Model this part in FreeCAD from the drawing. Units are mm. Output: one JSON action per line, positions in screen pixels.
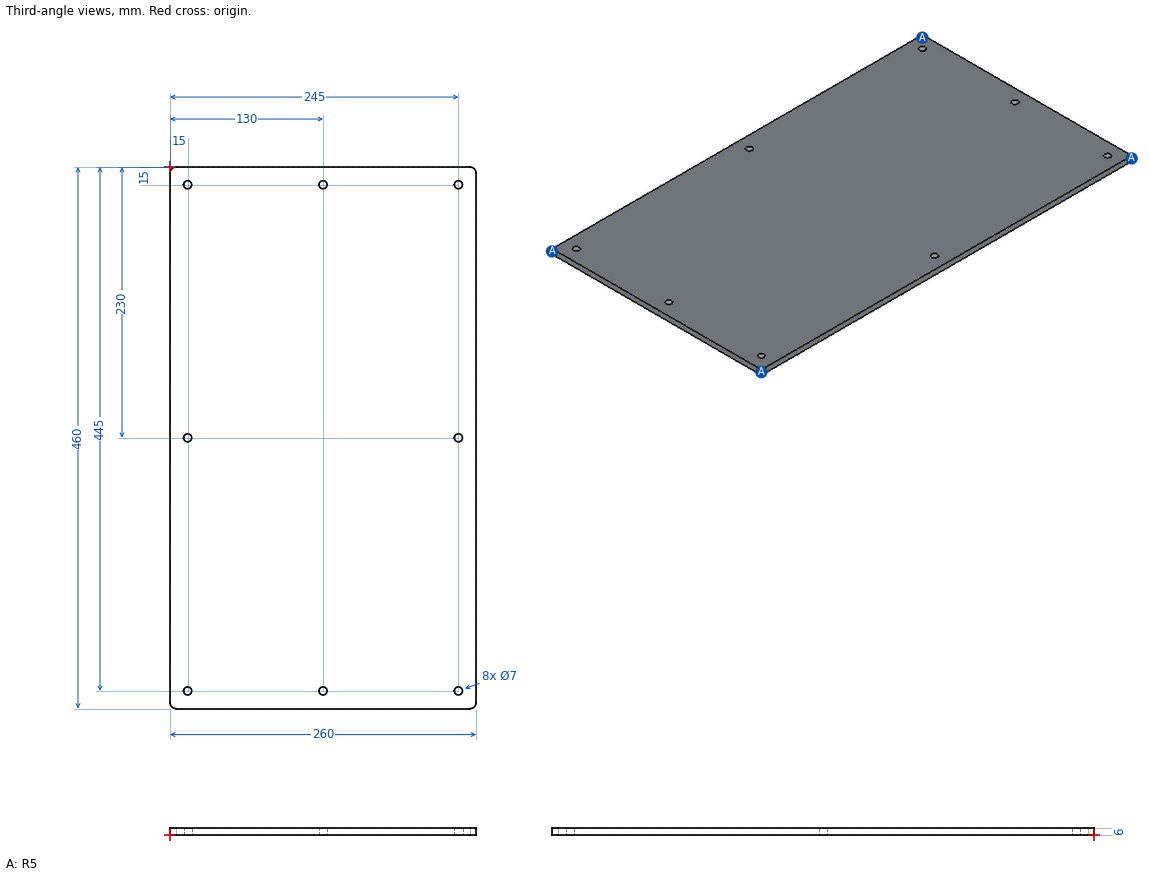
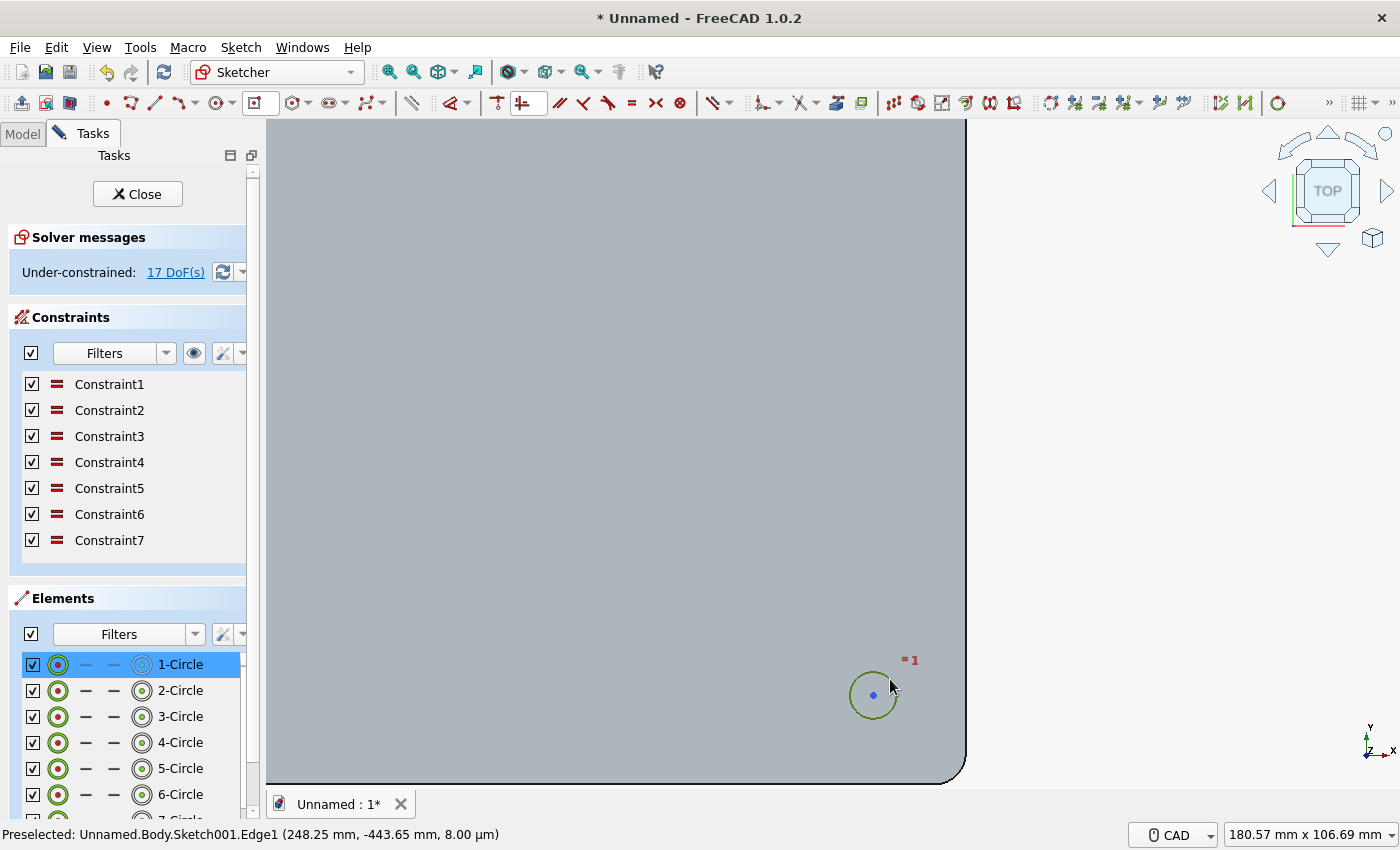
{"action": "key", "text": "k o"}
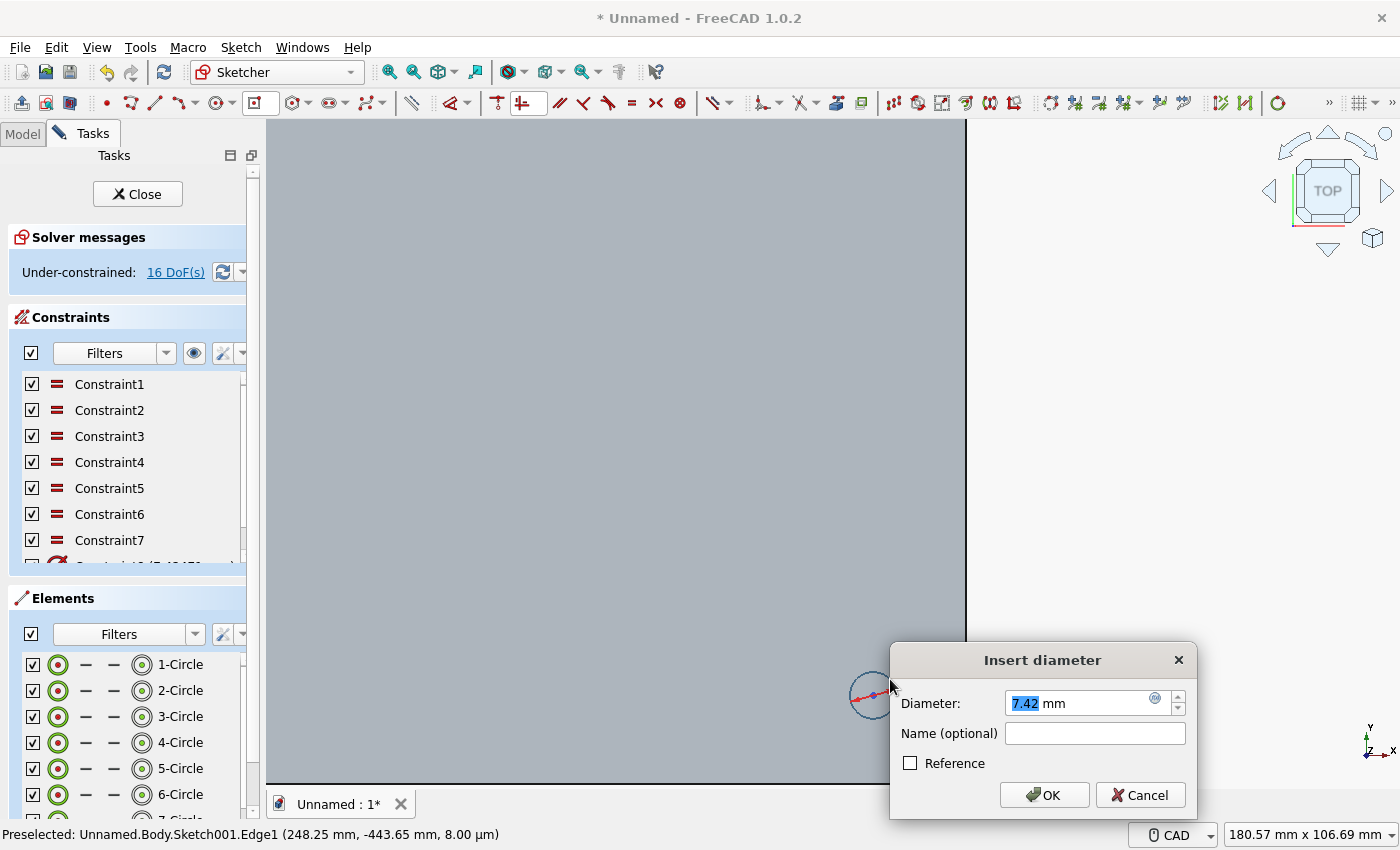
{"action": "type", "text": "7"}
{"action": "key", "text": "Return"}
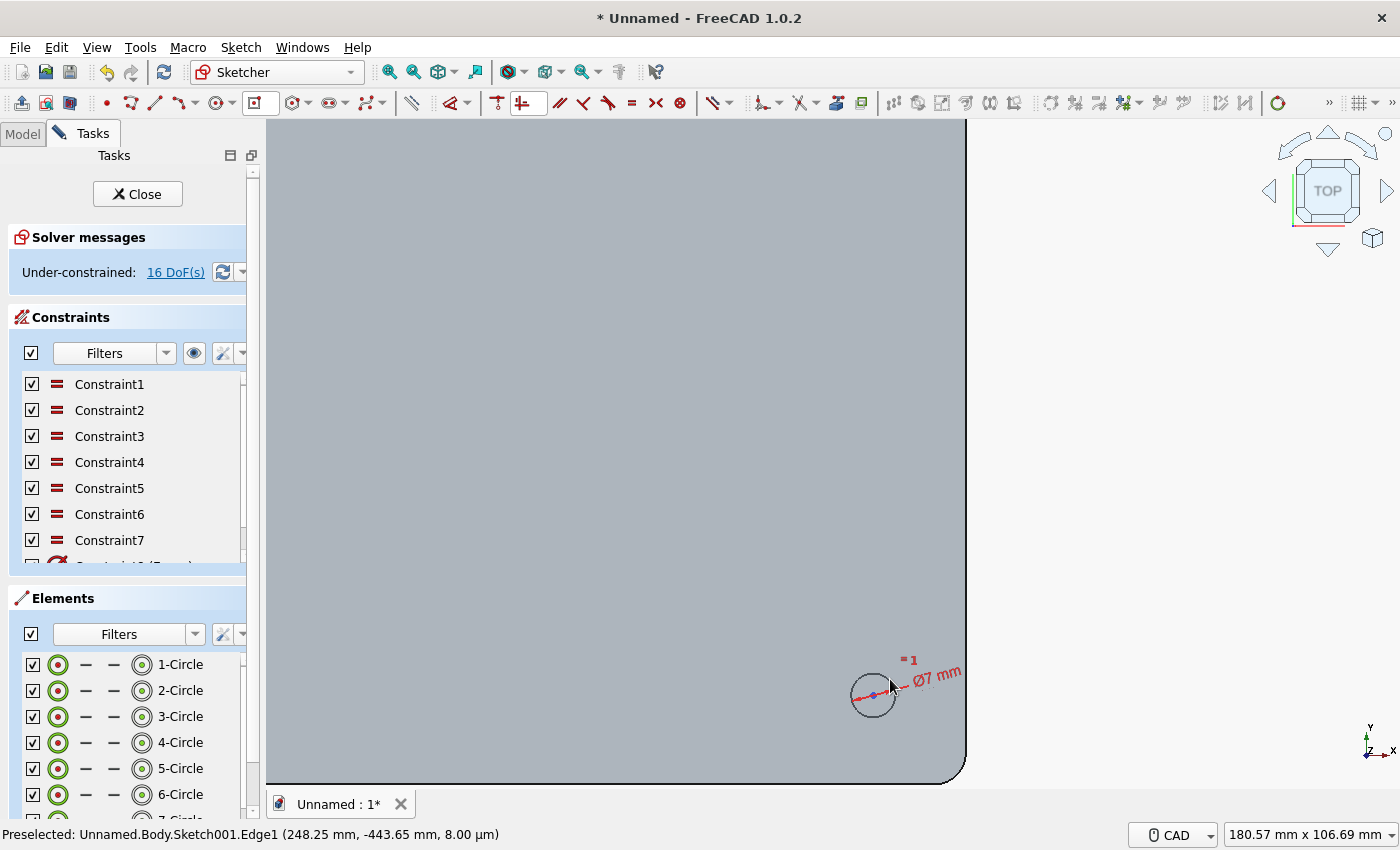
{"action": "scroll", "coordinate": [893, 682], "scroll_direction": "down", "scroll_amount": 9}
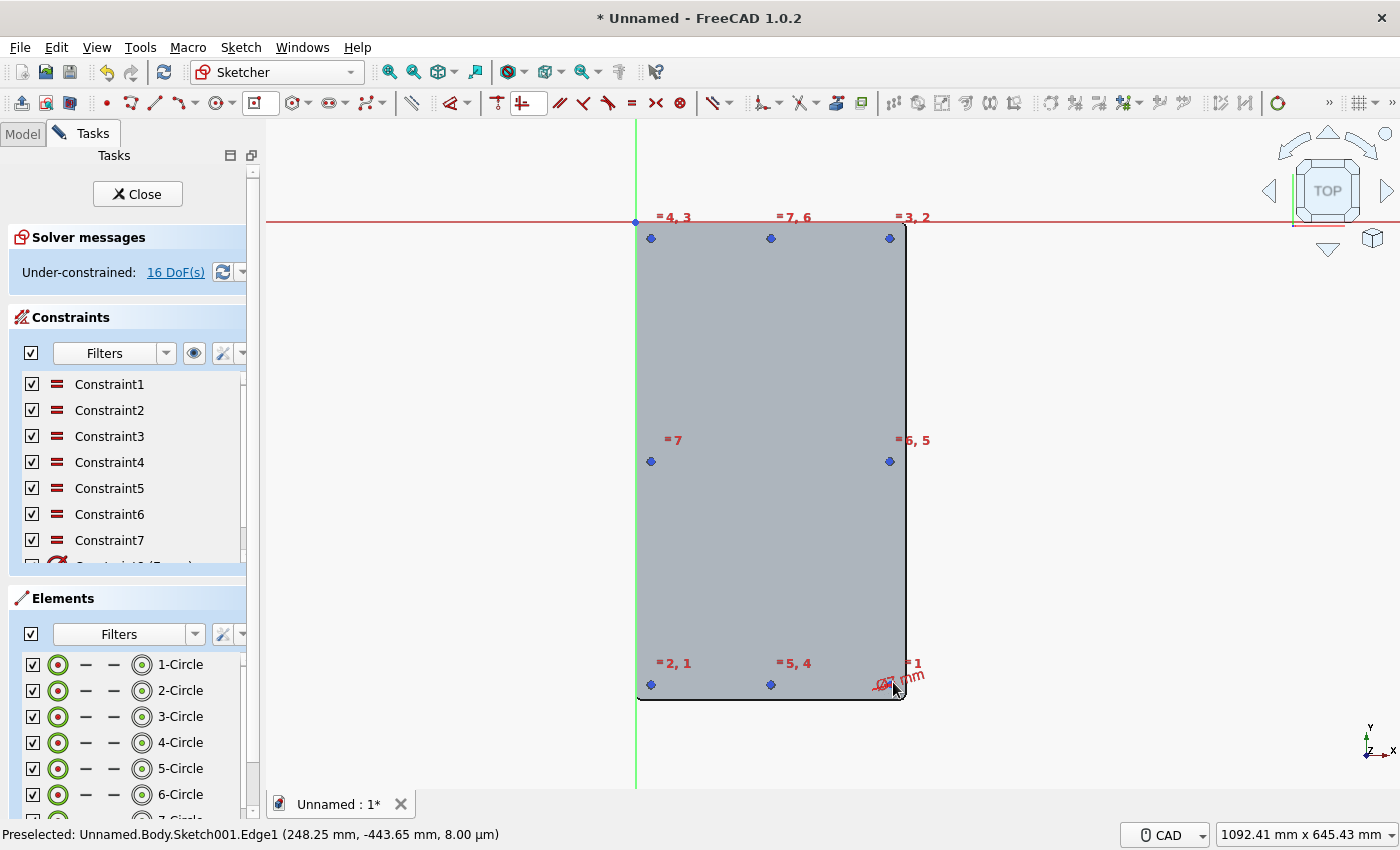
{"action": "scroll", "coordinate": [651, 685], "scroll_direction": "up", "scroll_amount": 5}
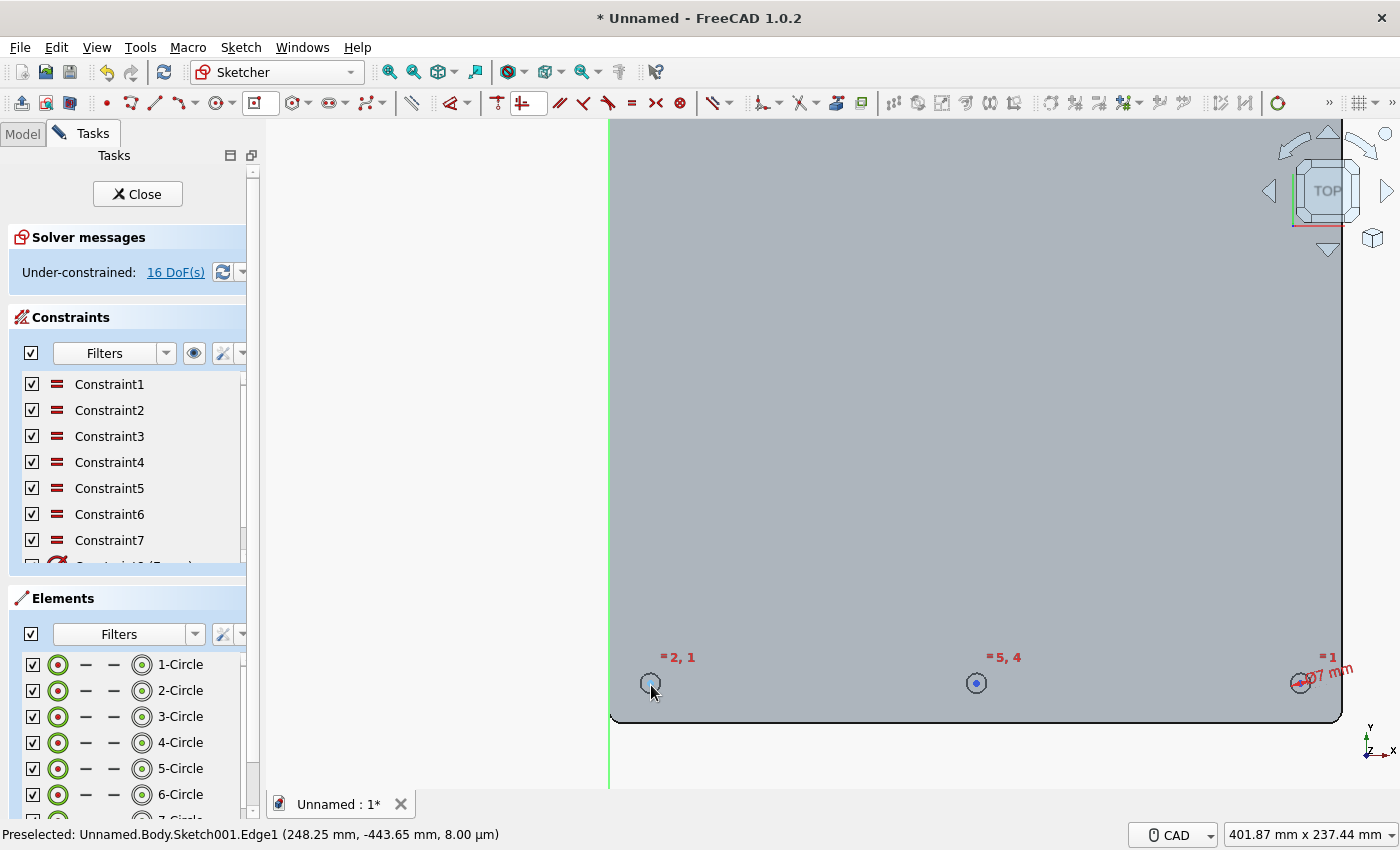
{"action": "left_click", "coordinate": [650, 683]}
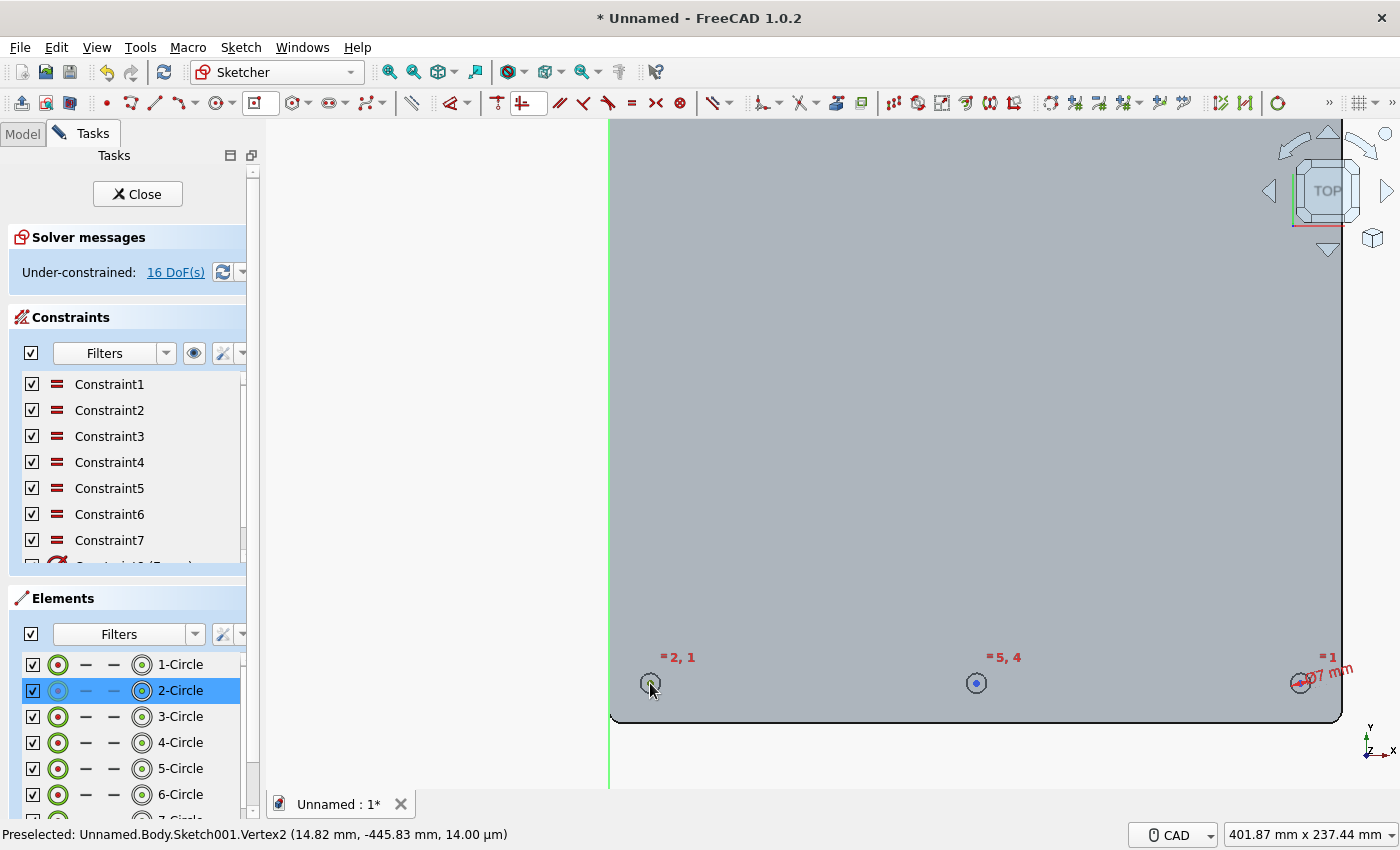
{"action": "left_click", "coordinate": [470, 104]}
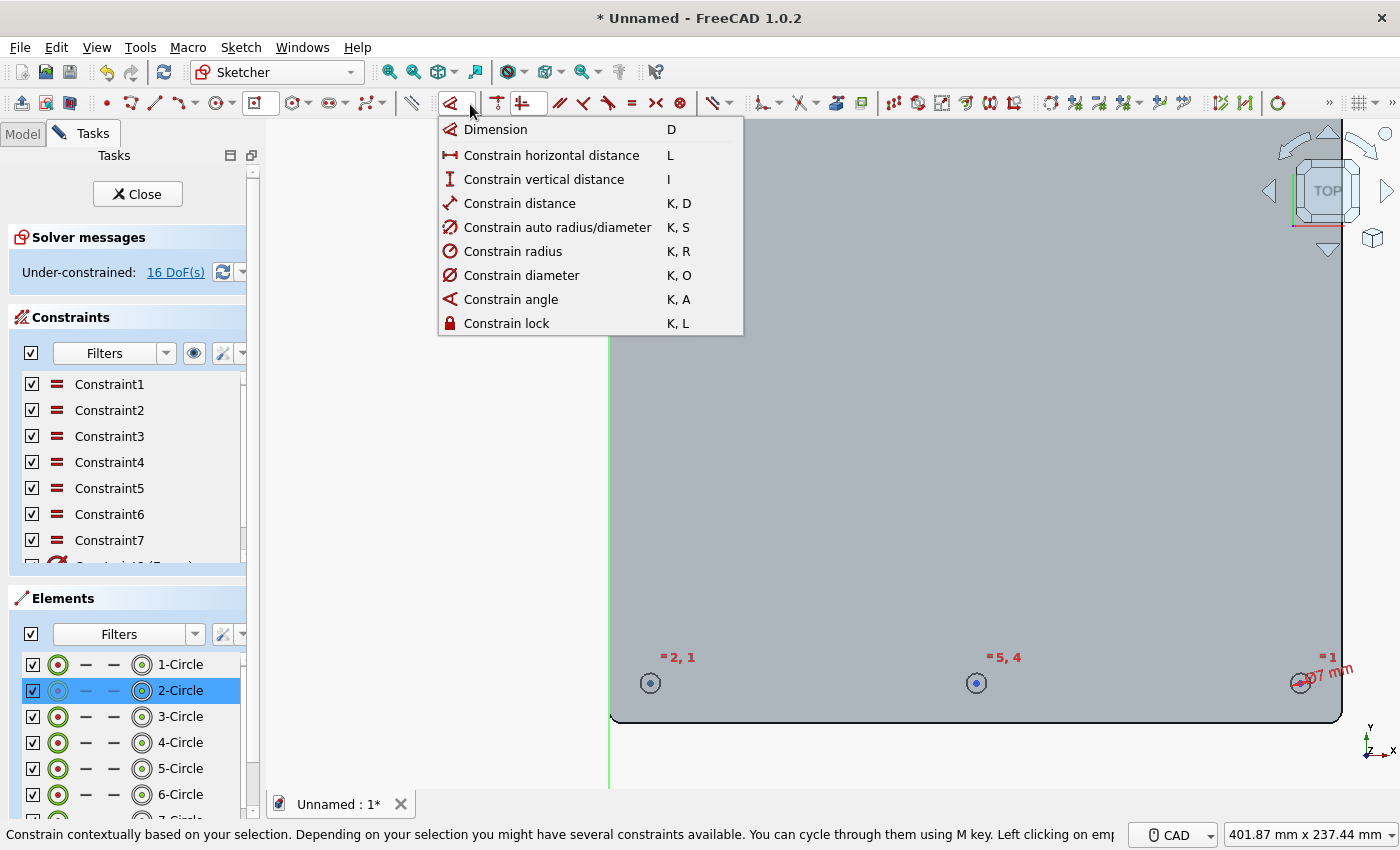
{"action": "left_click", "coordinate": [591, 155]}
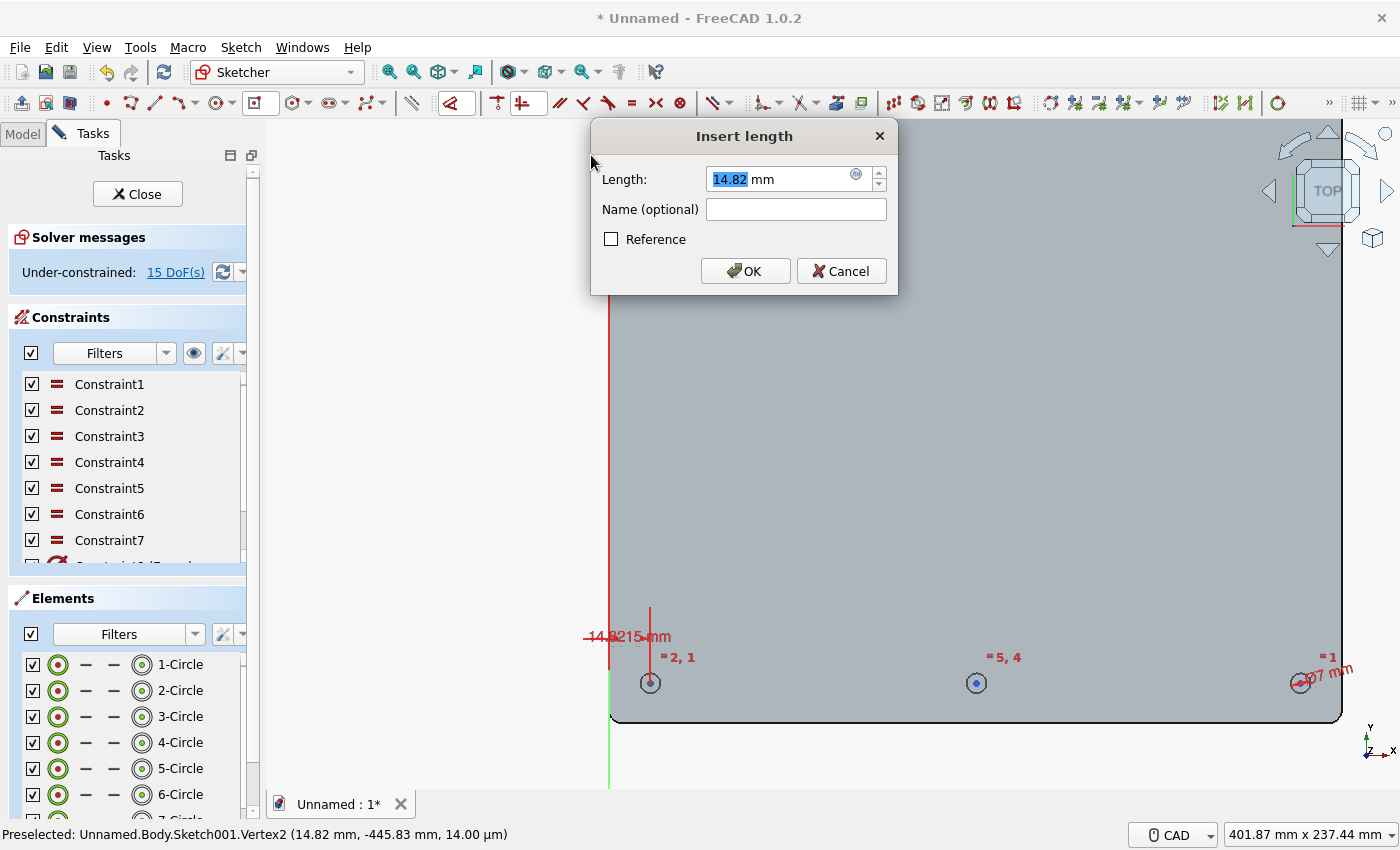
{"action": "type", "text": "15"}
{"action": "key", "text": "Return"}